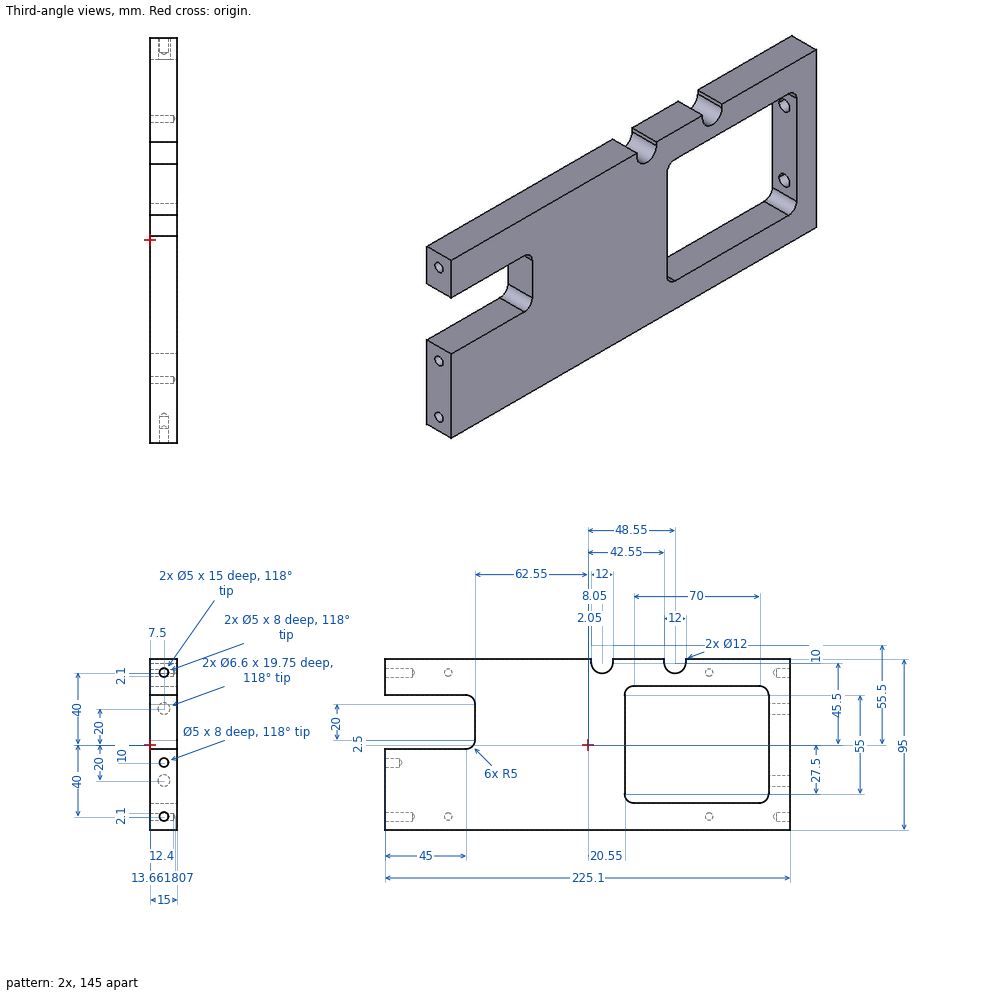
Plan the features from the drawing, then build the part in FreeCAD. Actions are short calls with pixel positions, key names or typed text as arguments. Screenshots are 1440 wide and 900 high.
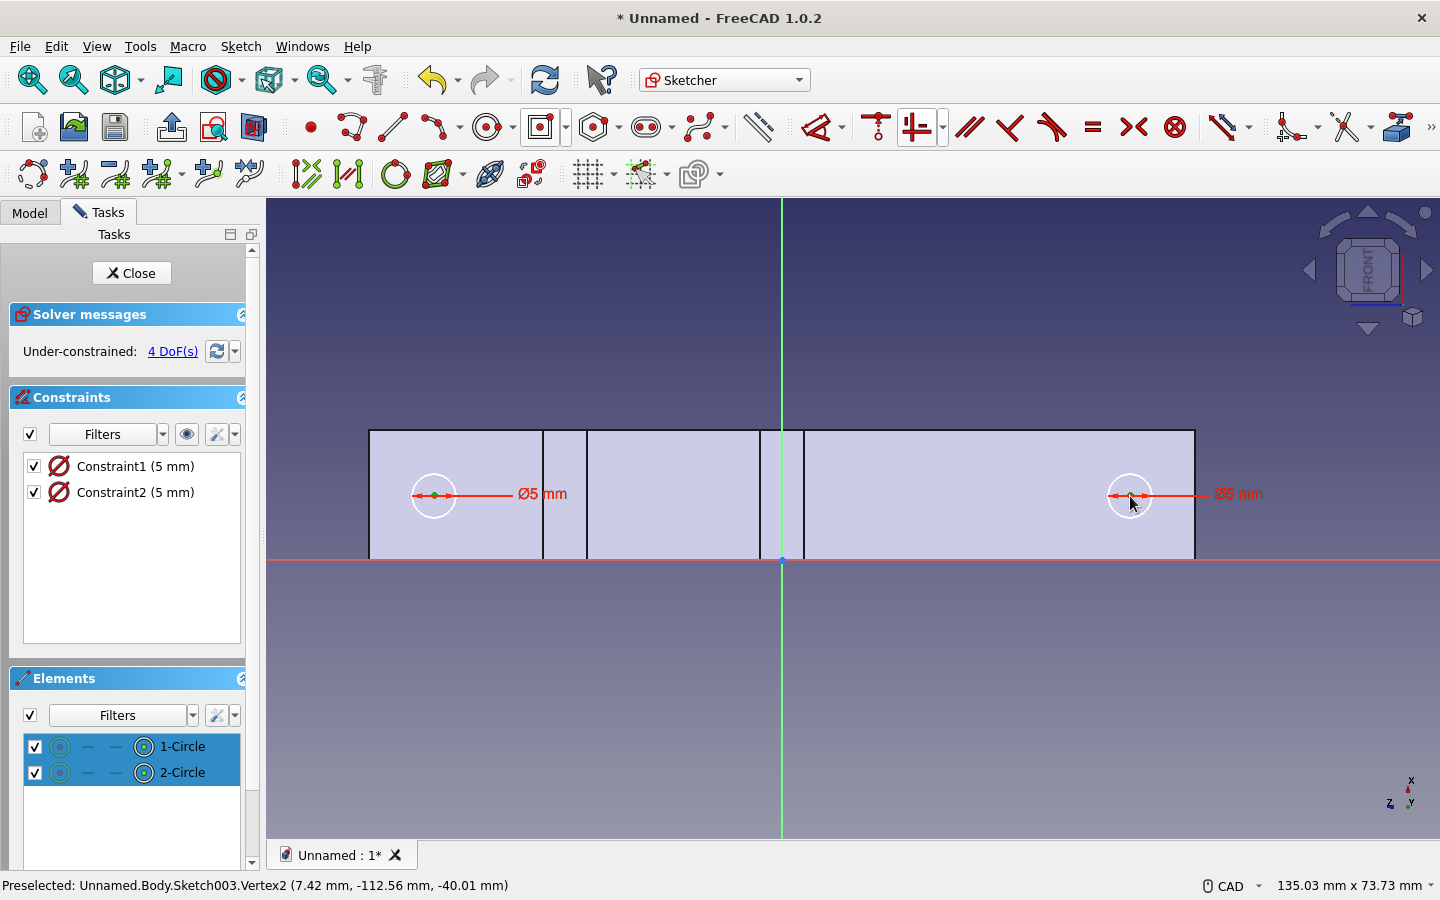
key(h)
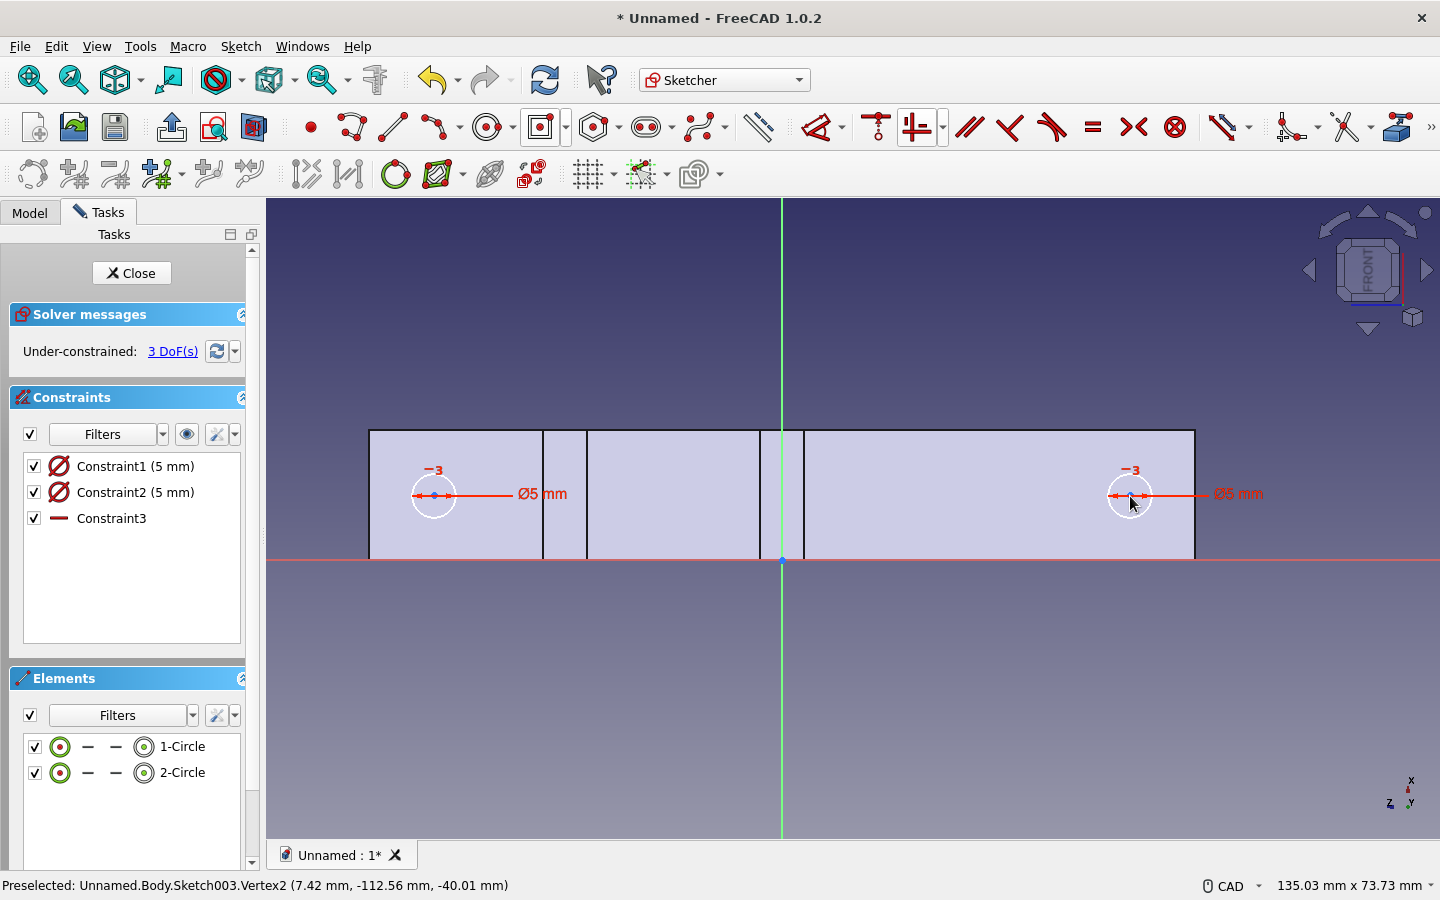
click(816, 128)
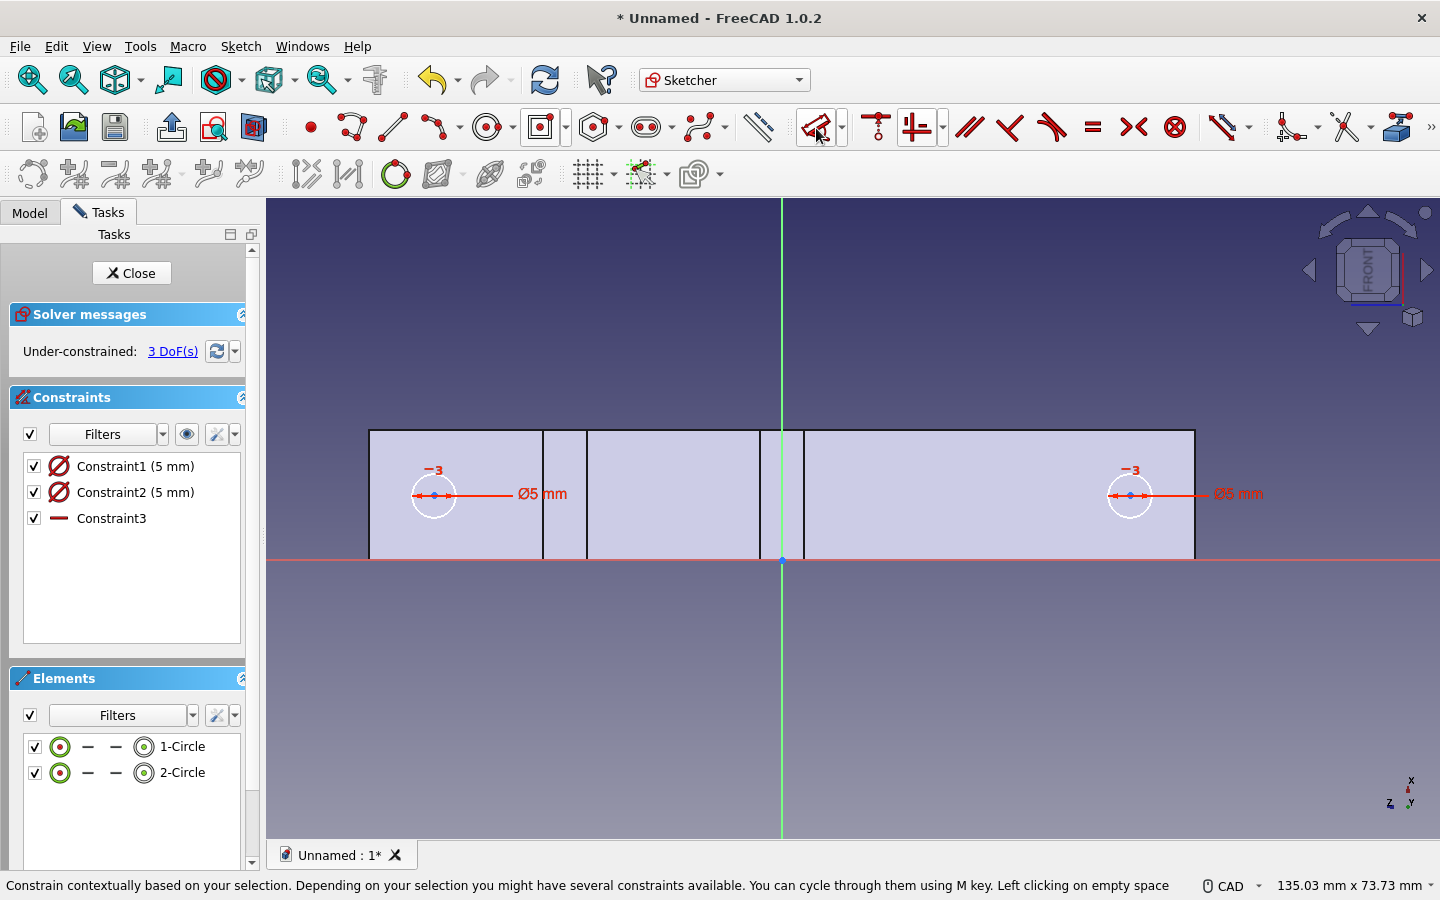
click(434, 496)
click(608, 594)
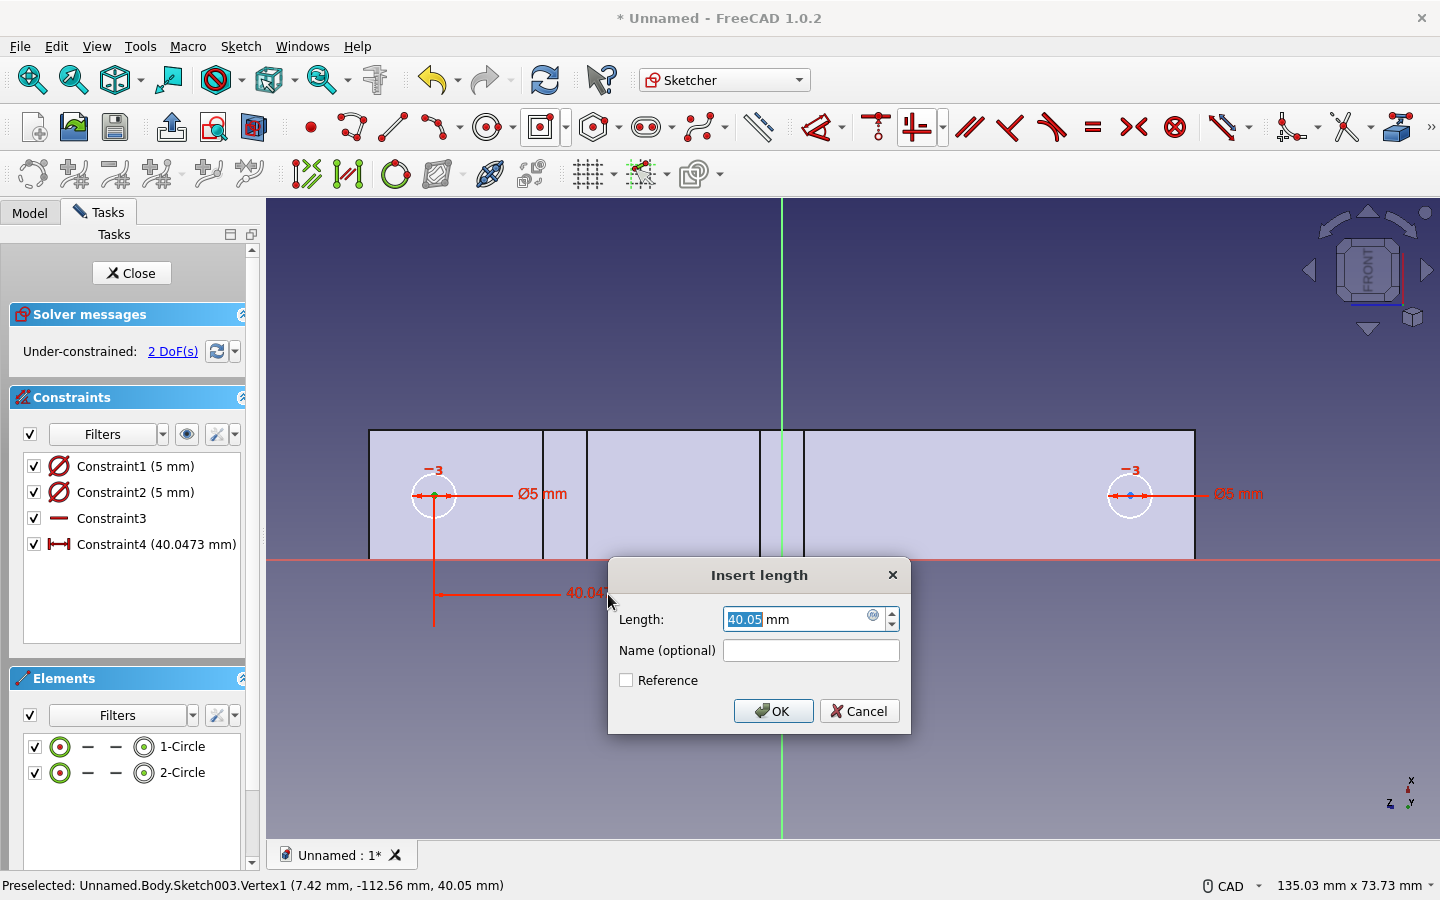
text(40)
key(Return)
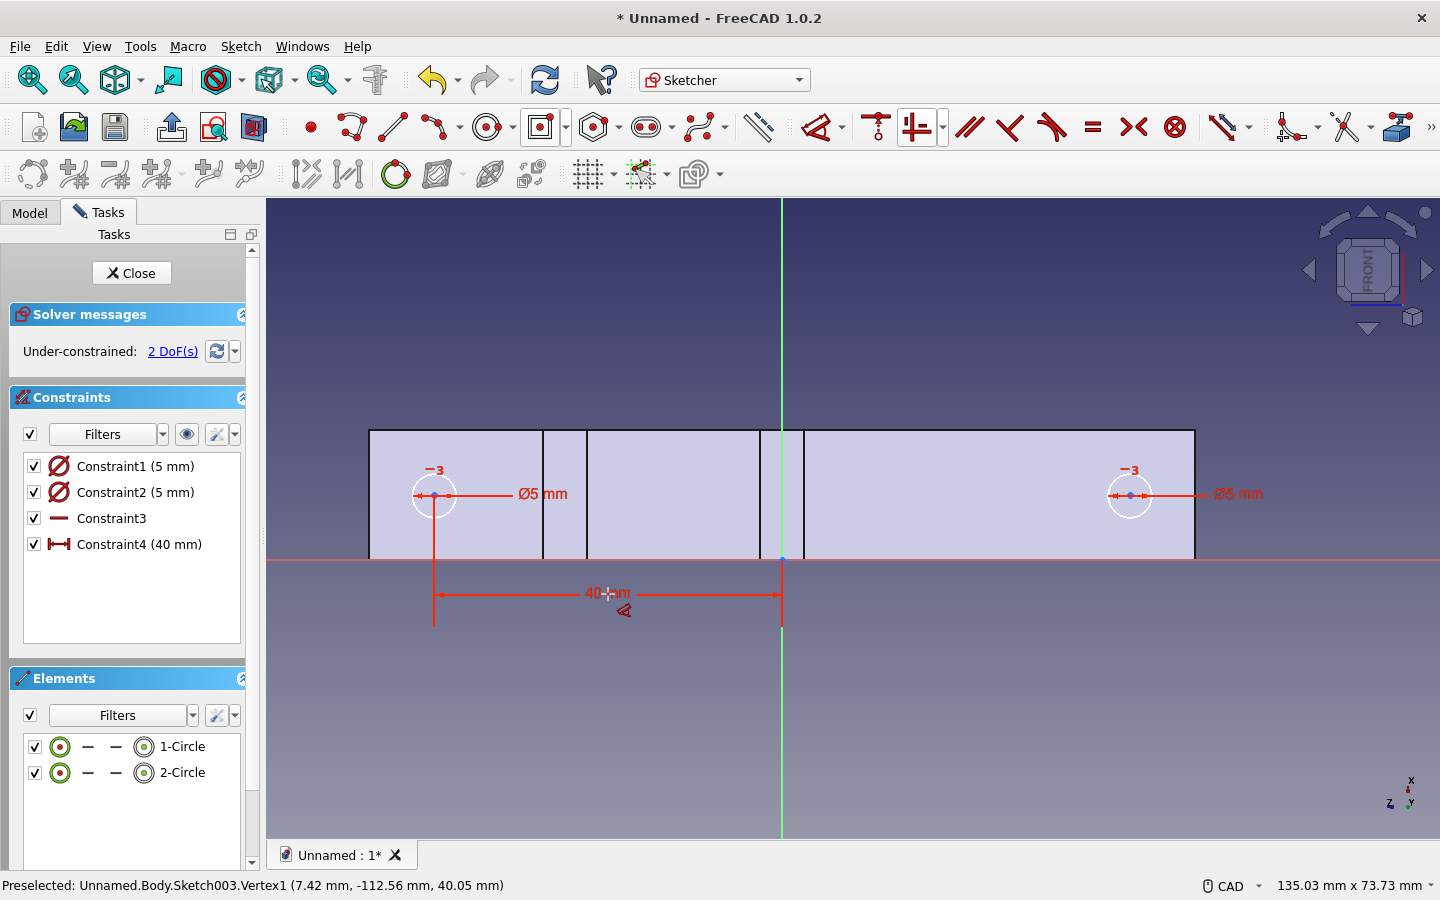
click(1130, 496)
click(956, 594)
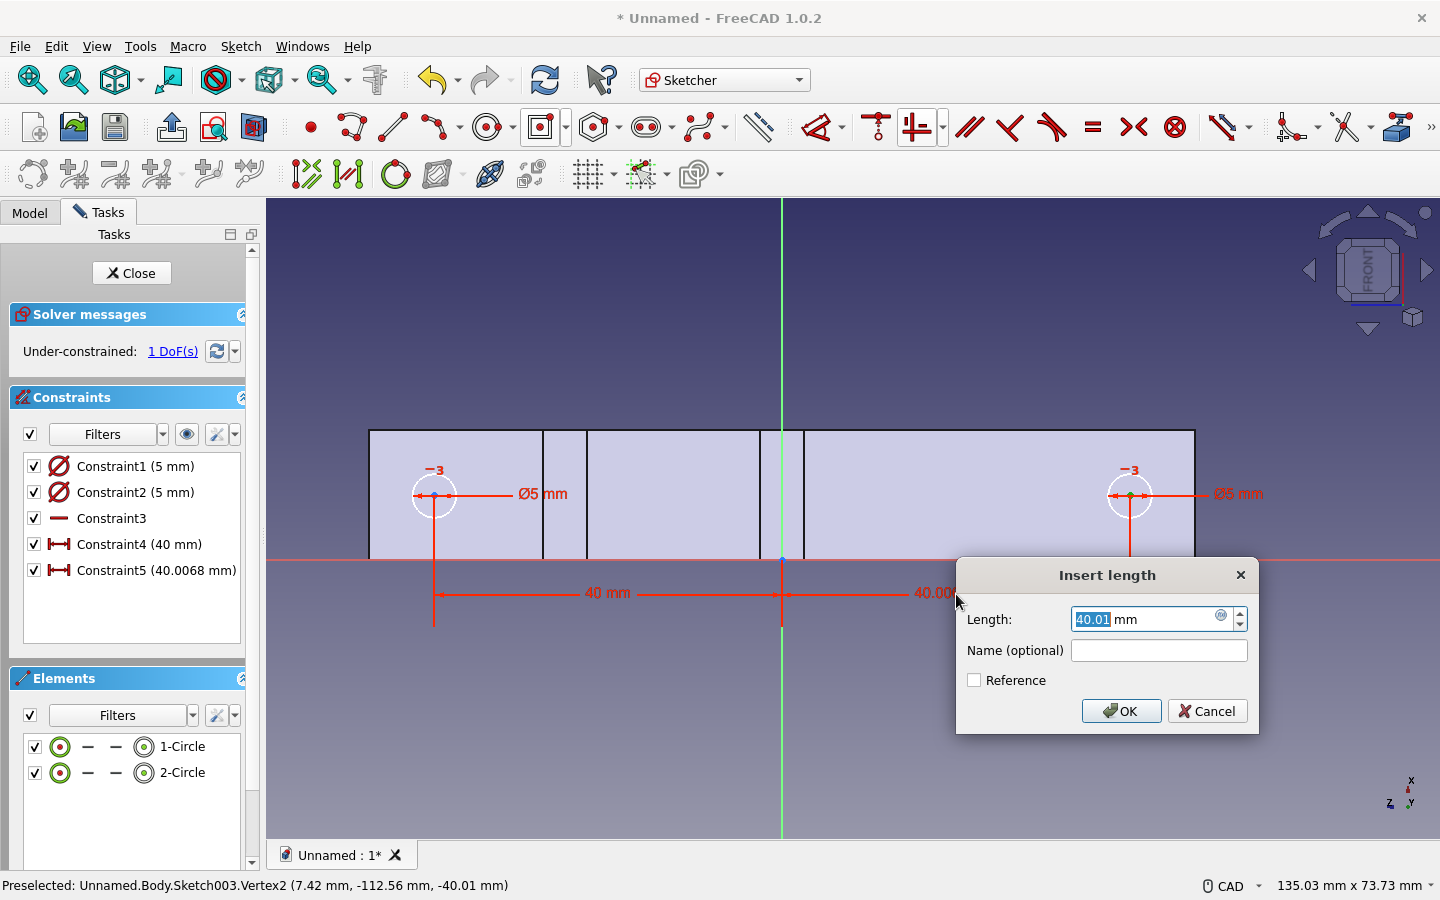
text(40)
key(Return)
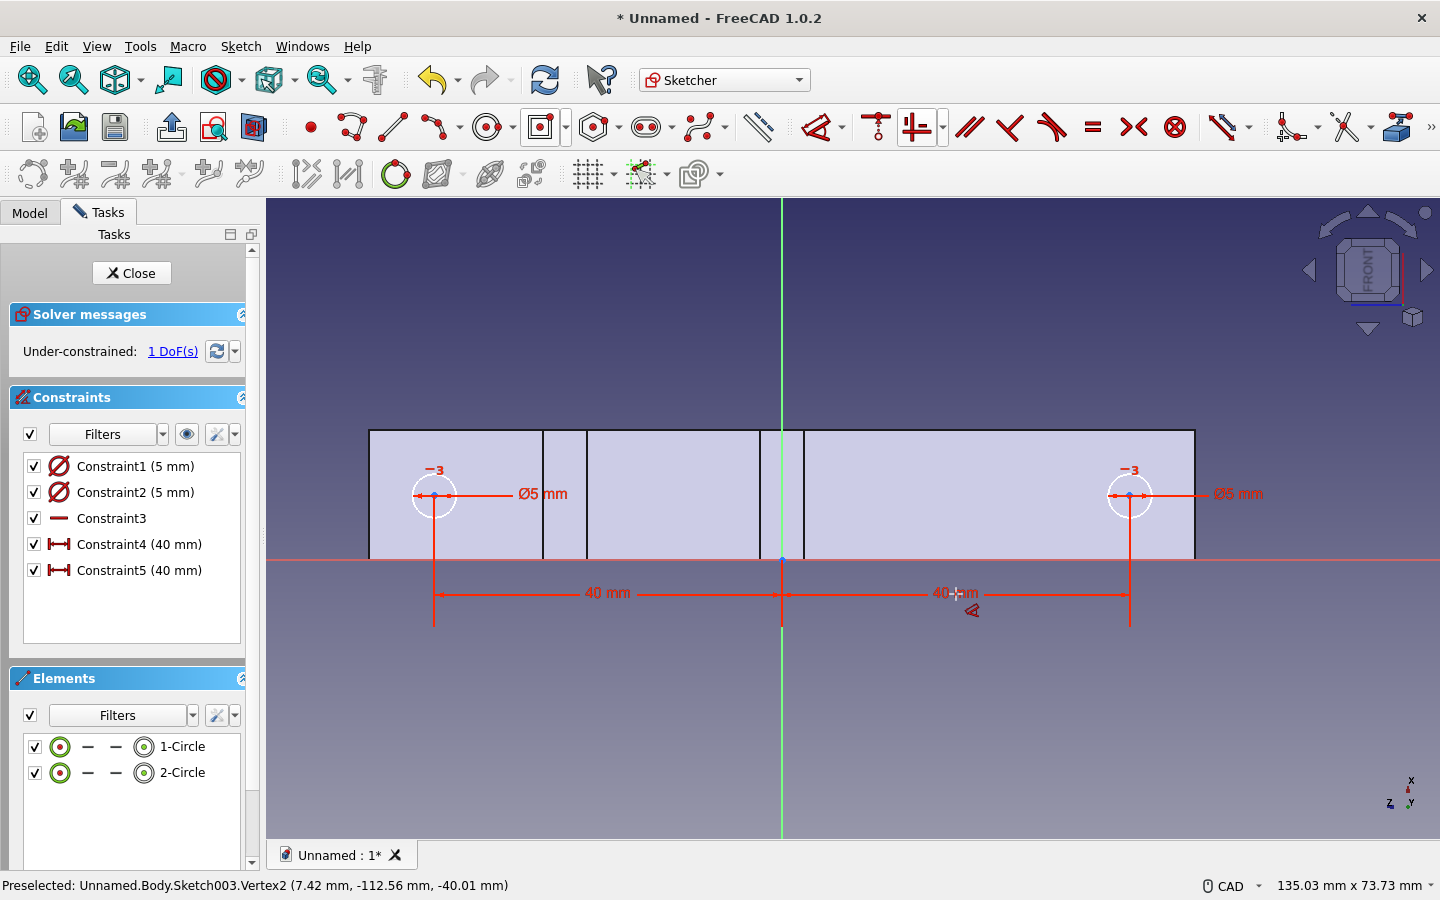
click(434, 496)
click(400, 528)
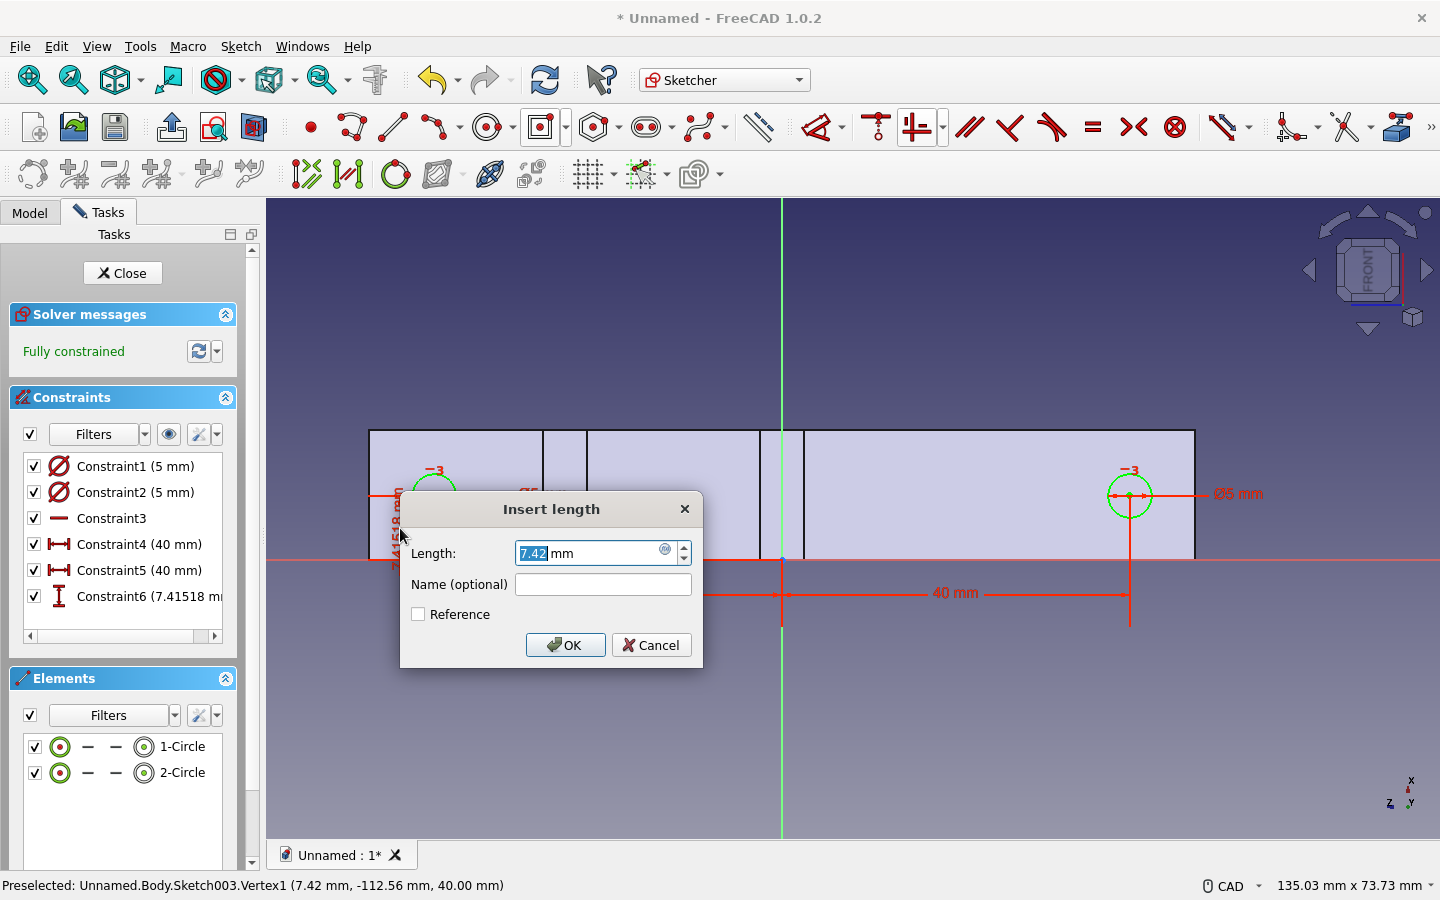
text(7.5)
key(Return)
key(Escape)